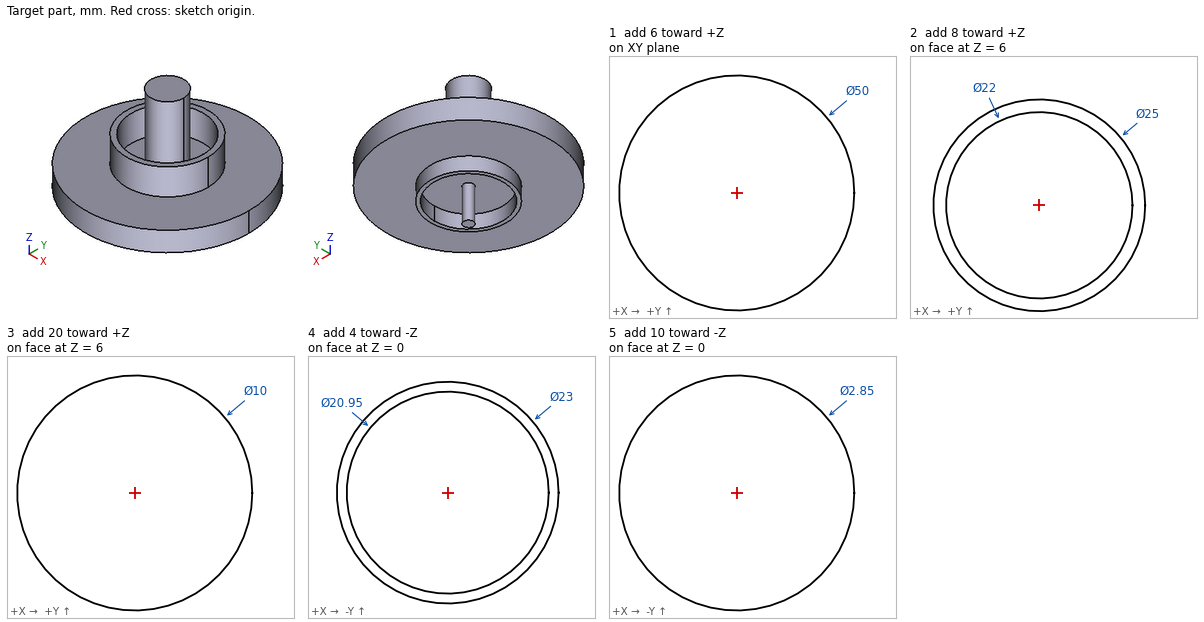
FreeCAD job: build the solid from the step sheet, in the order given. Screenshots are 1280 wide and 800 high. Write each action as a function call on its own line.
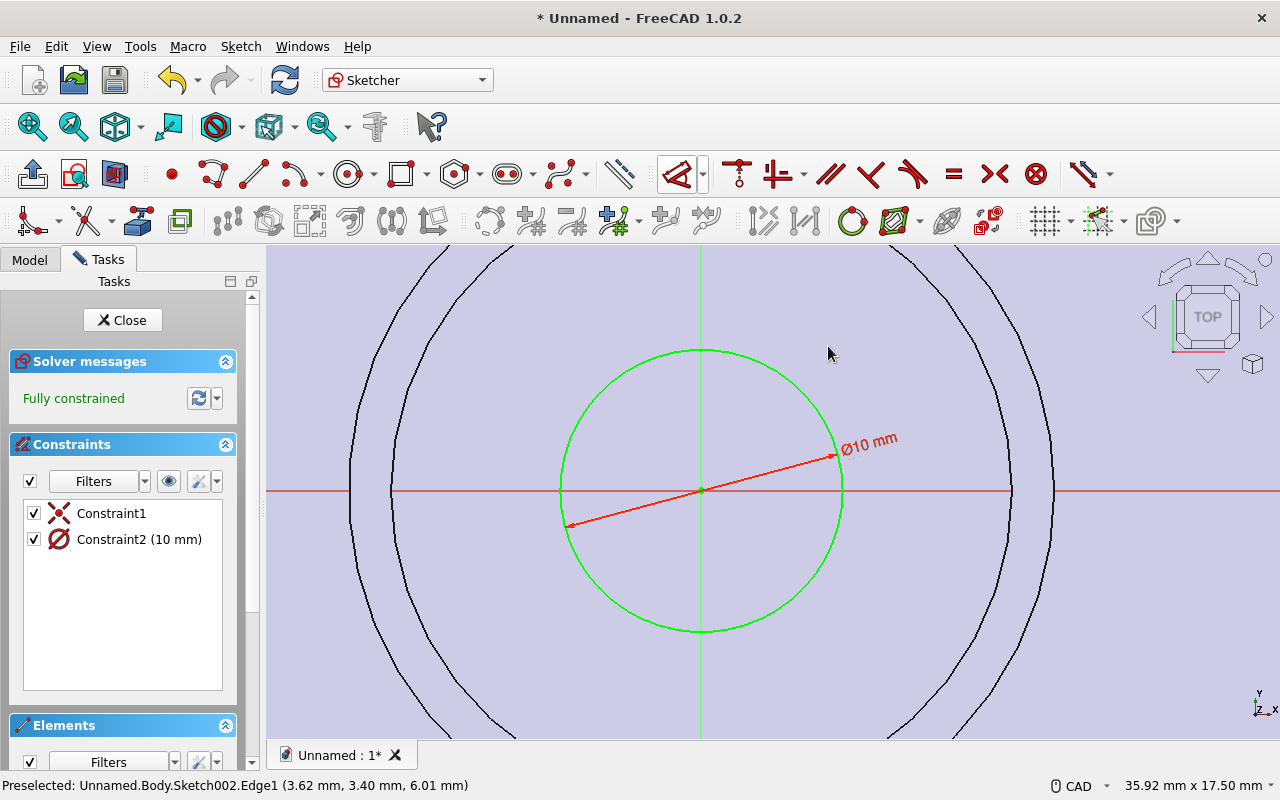
click(123, 320)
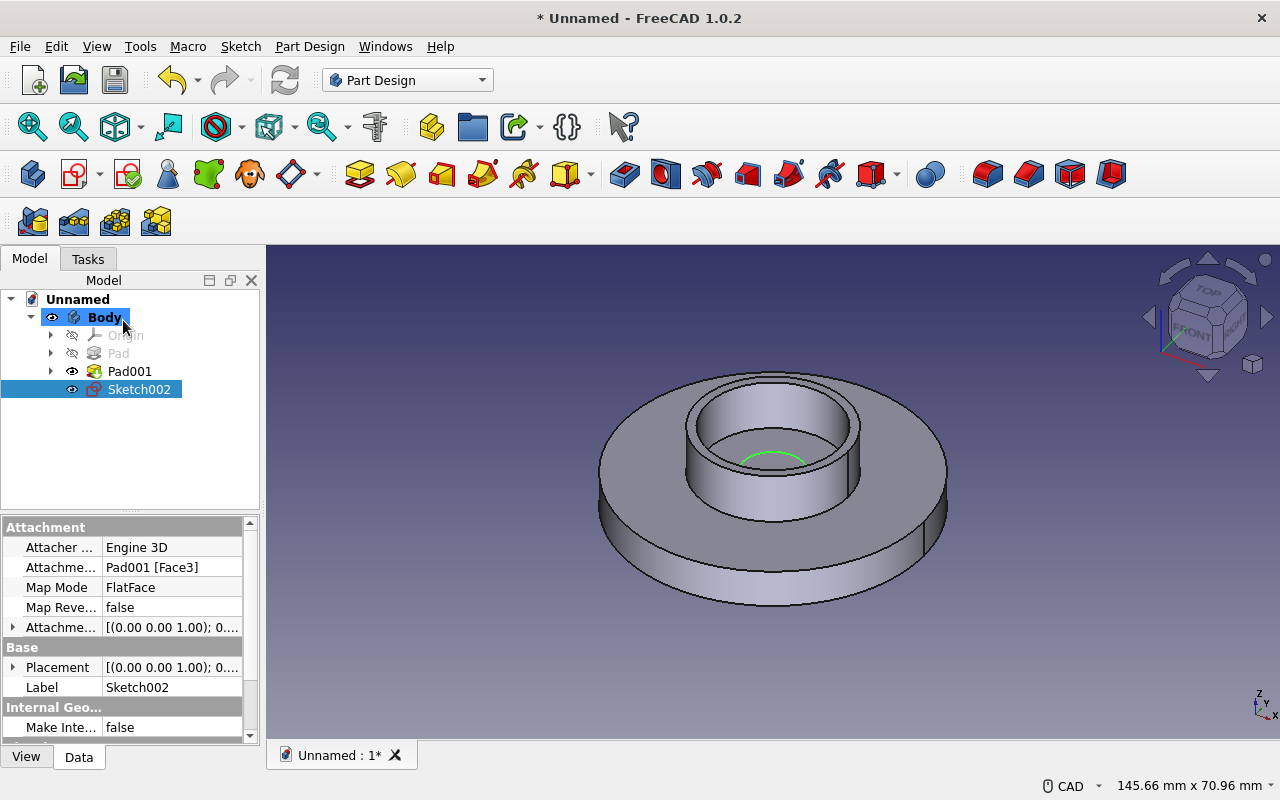
click(360, 174)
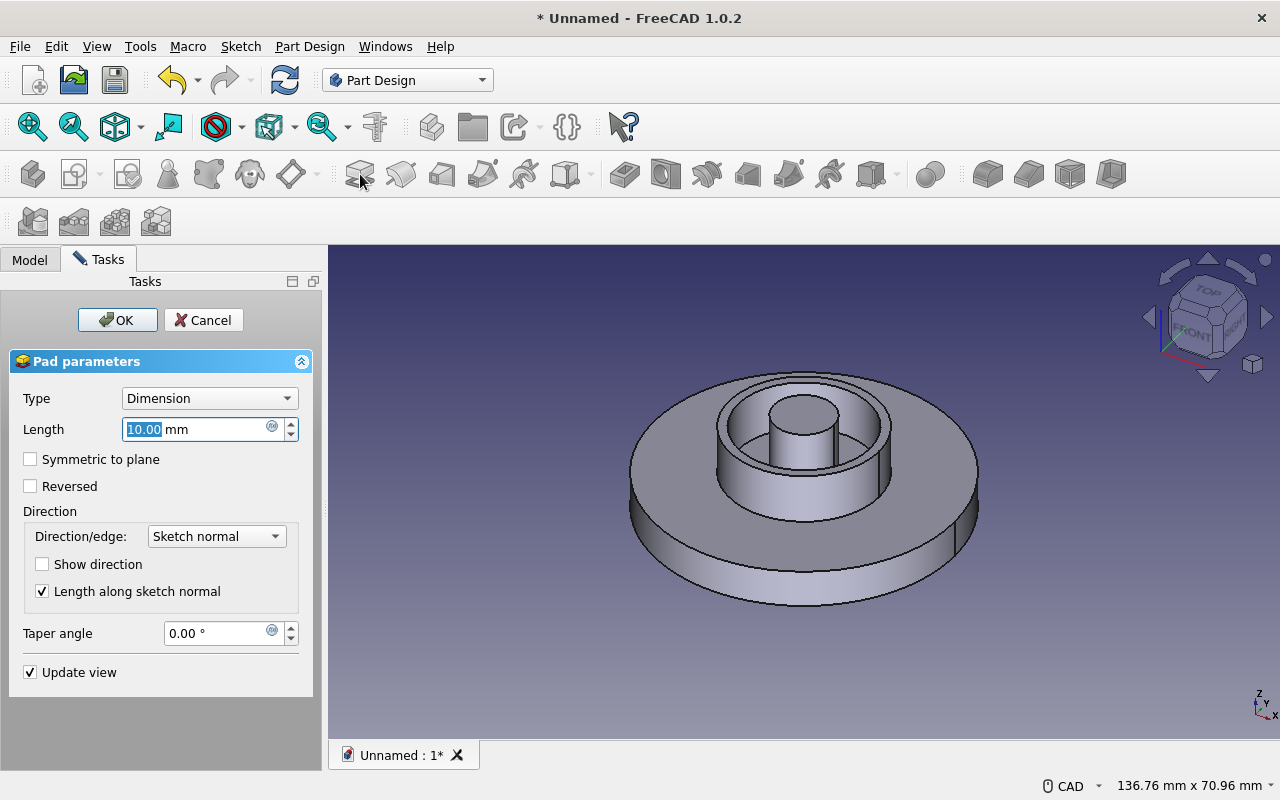
text(20)
key(Tab)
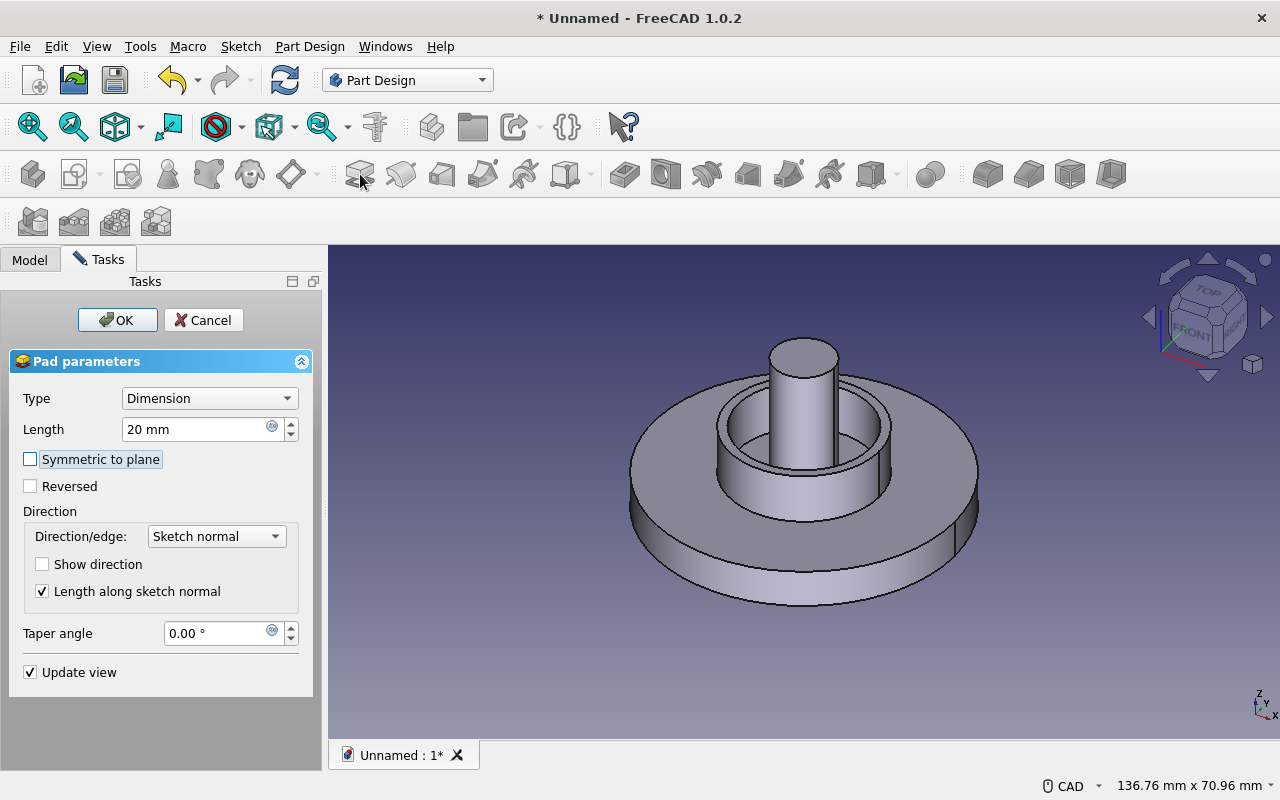
click(118, 320)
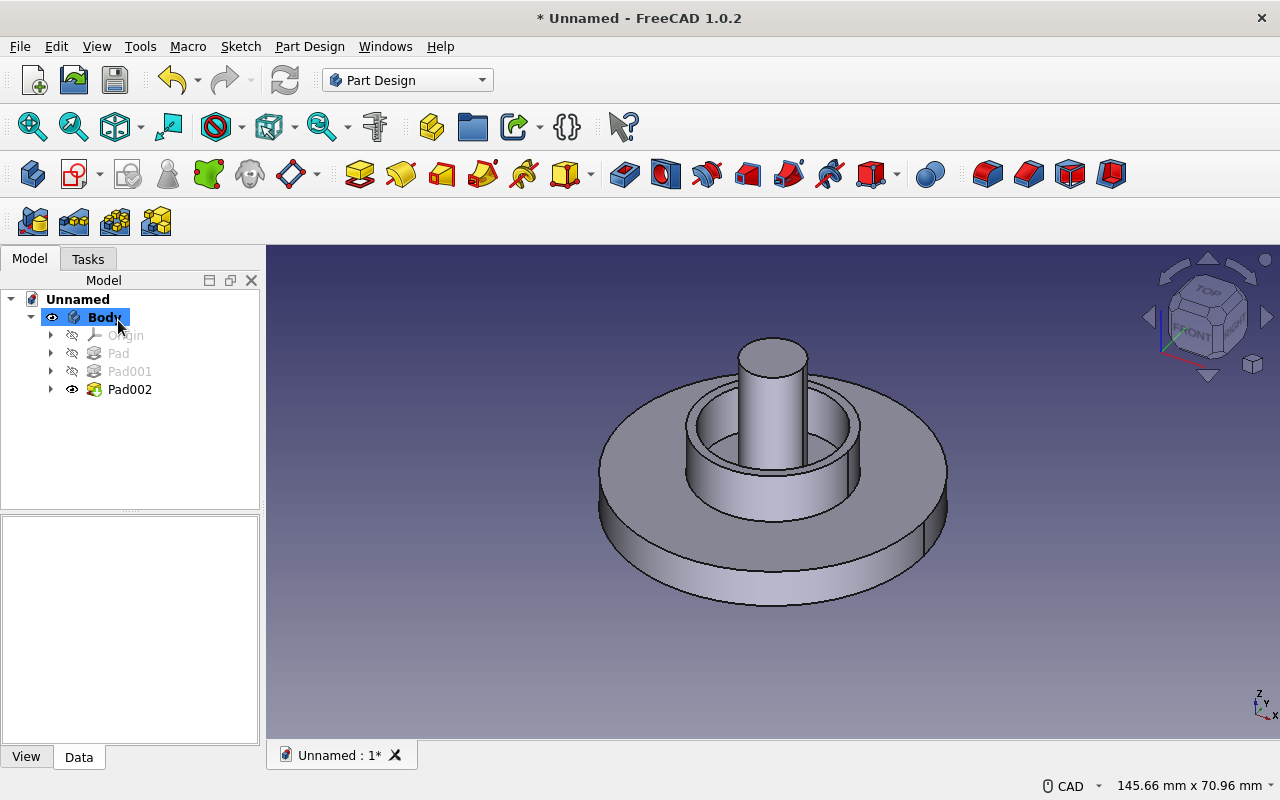
click(33, 128)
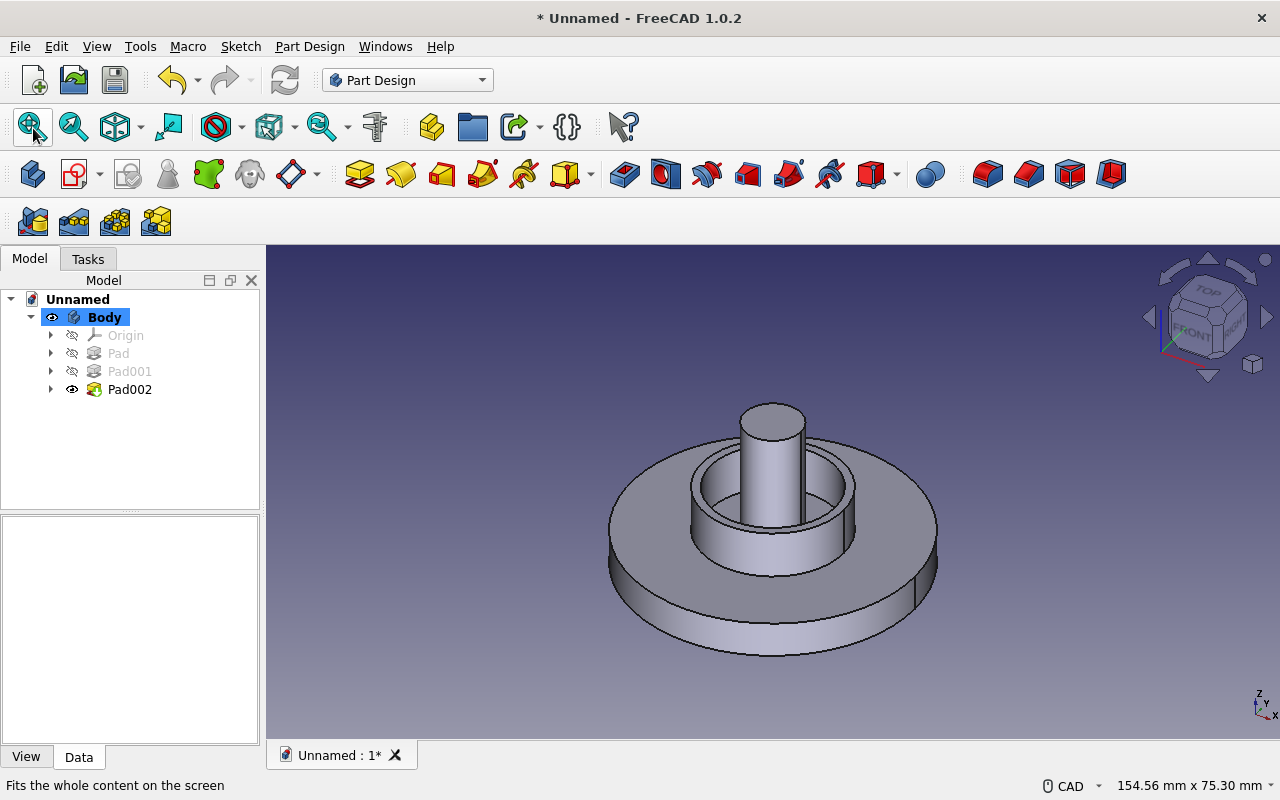
key(5)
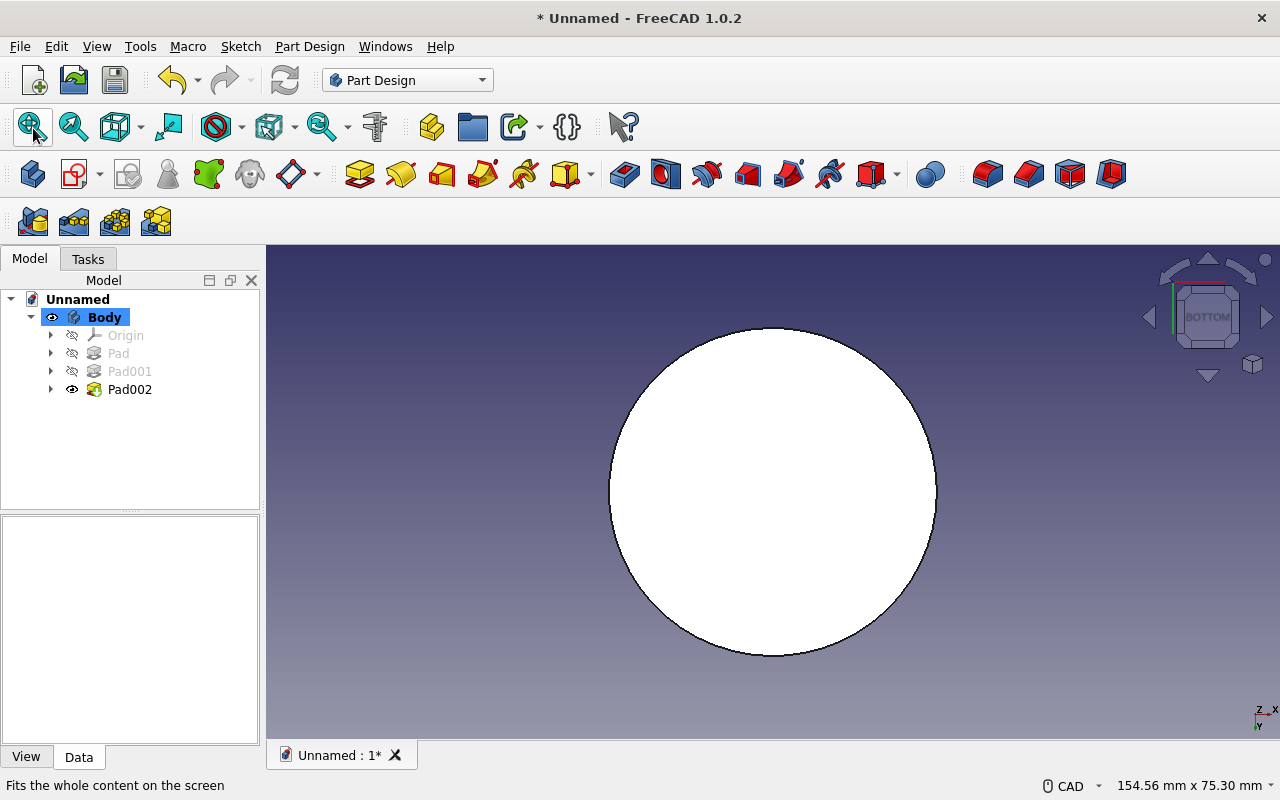
click(773, 491)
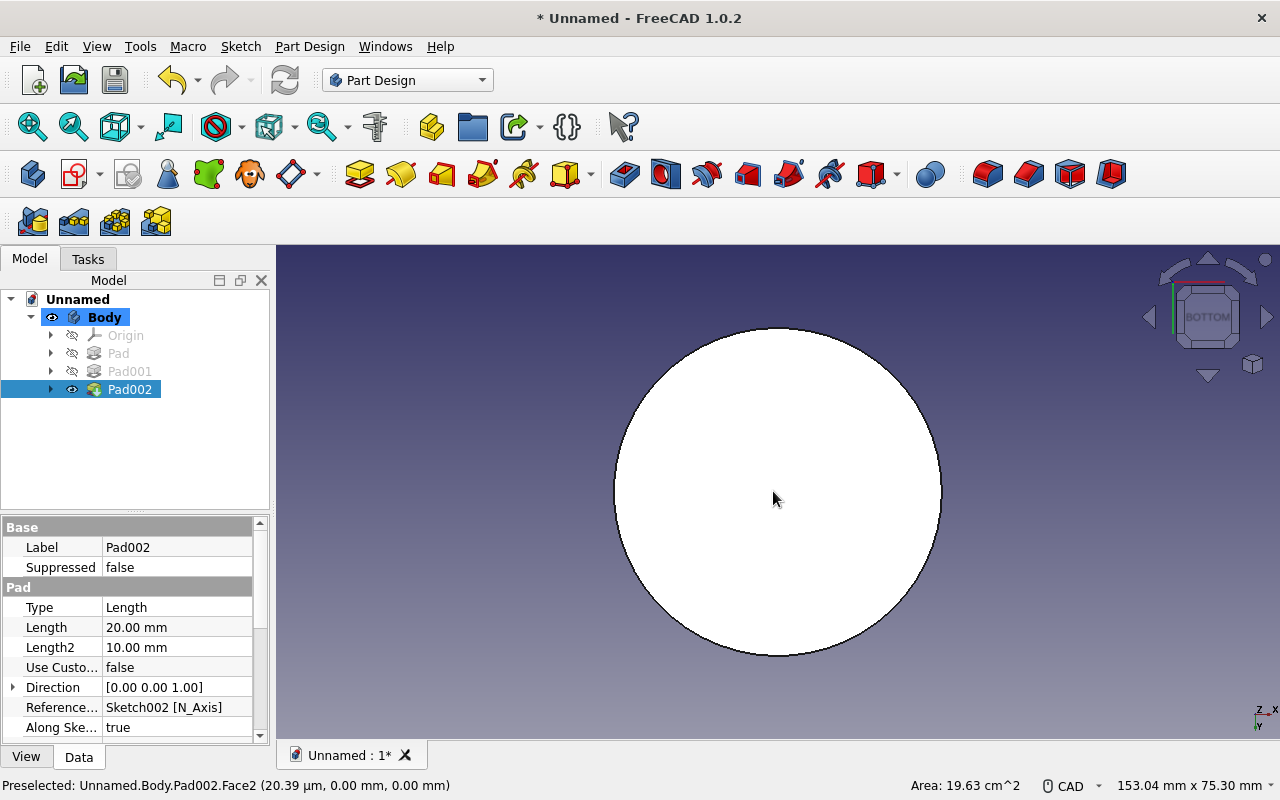
click(74, 174)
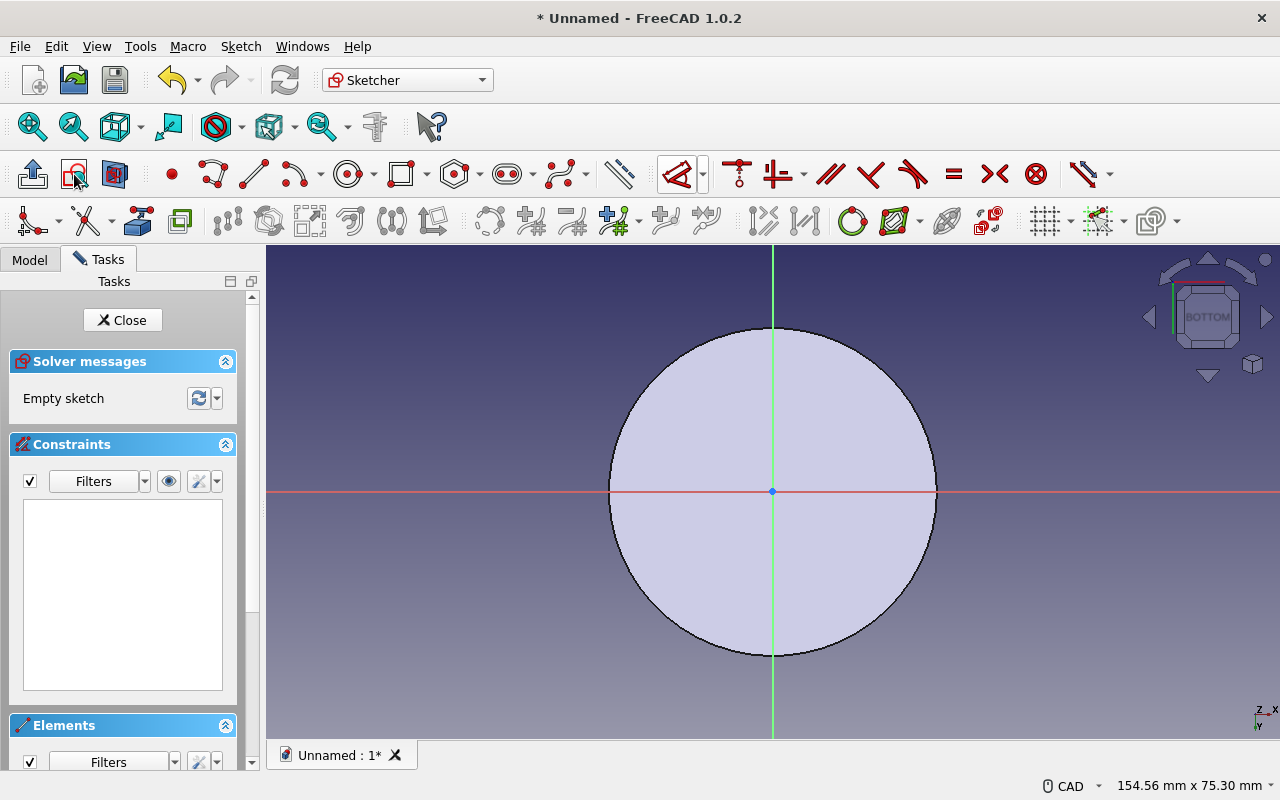
scroll(829, 492, up, 4)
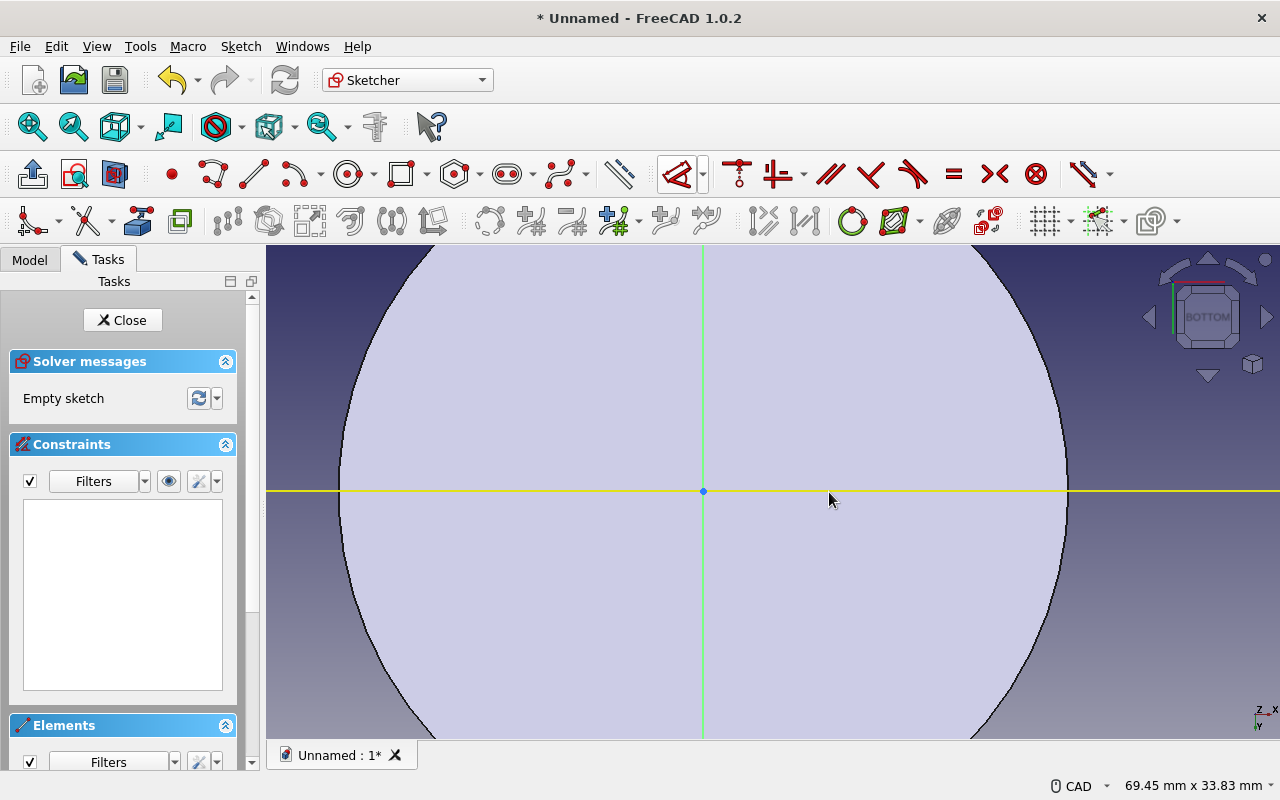
click(348, 174)